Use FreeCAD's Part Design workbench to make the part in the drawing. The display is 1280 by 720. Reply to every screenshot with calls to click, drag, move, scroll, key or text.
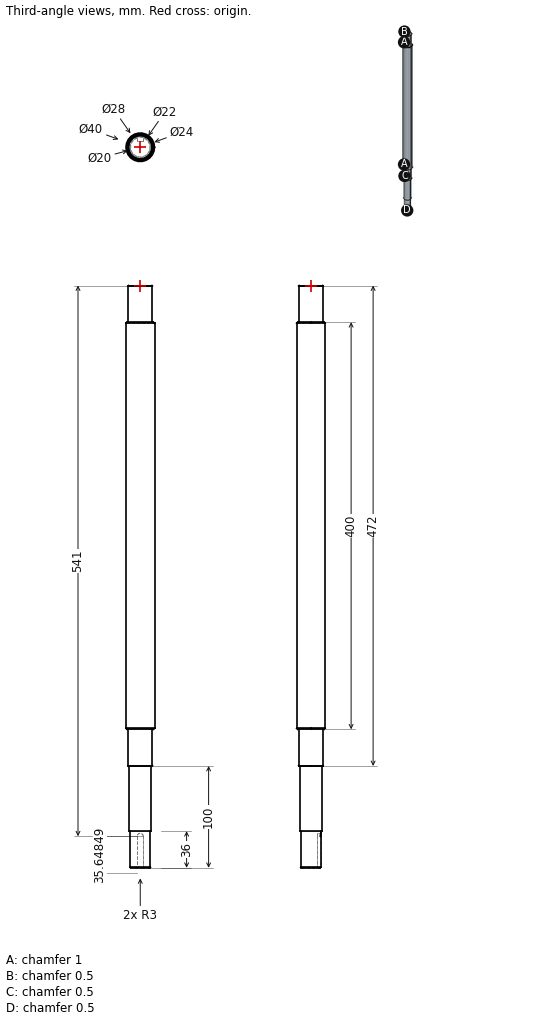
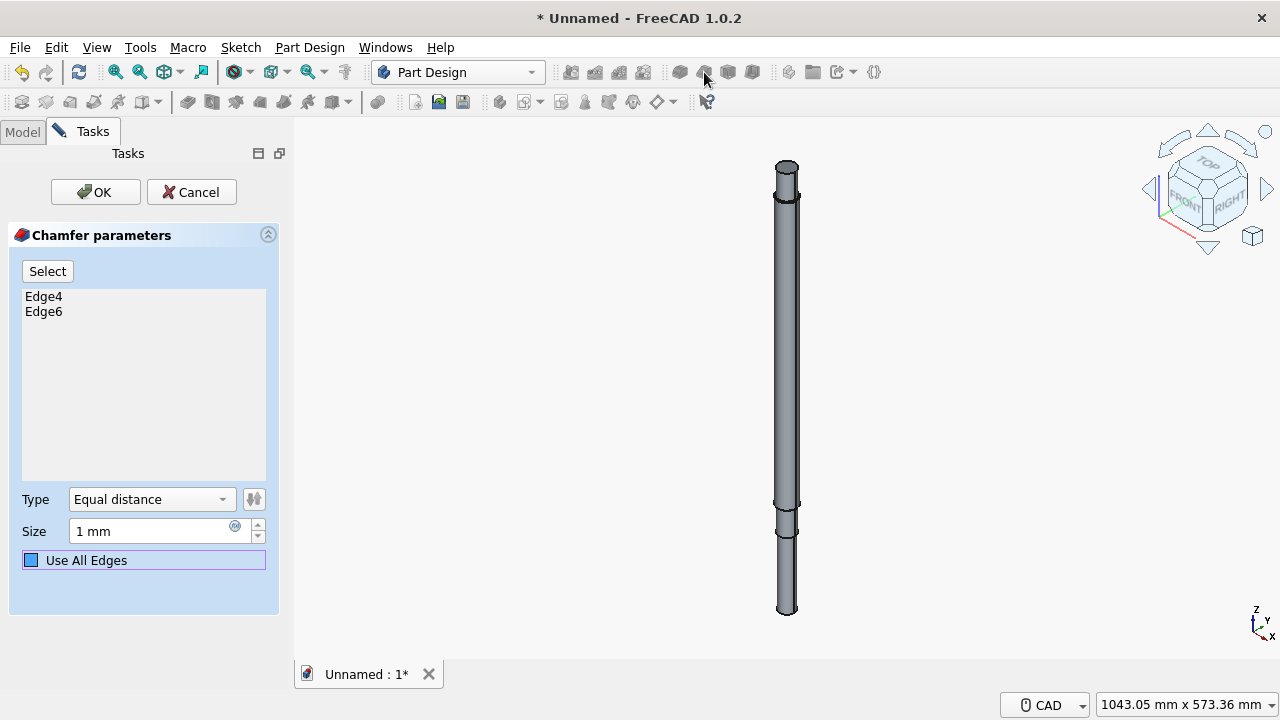
click(96, 192)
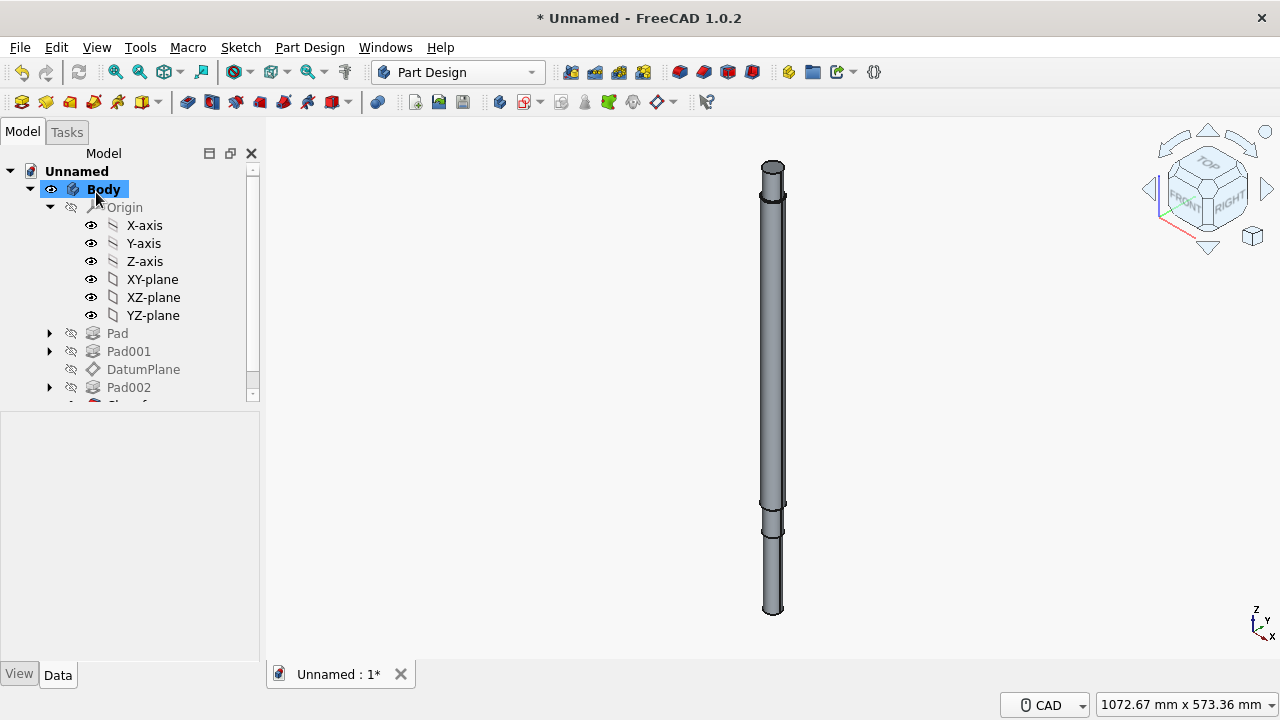
click(762, 165)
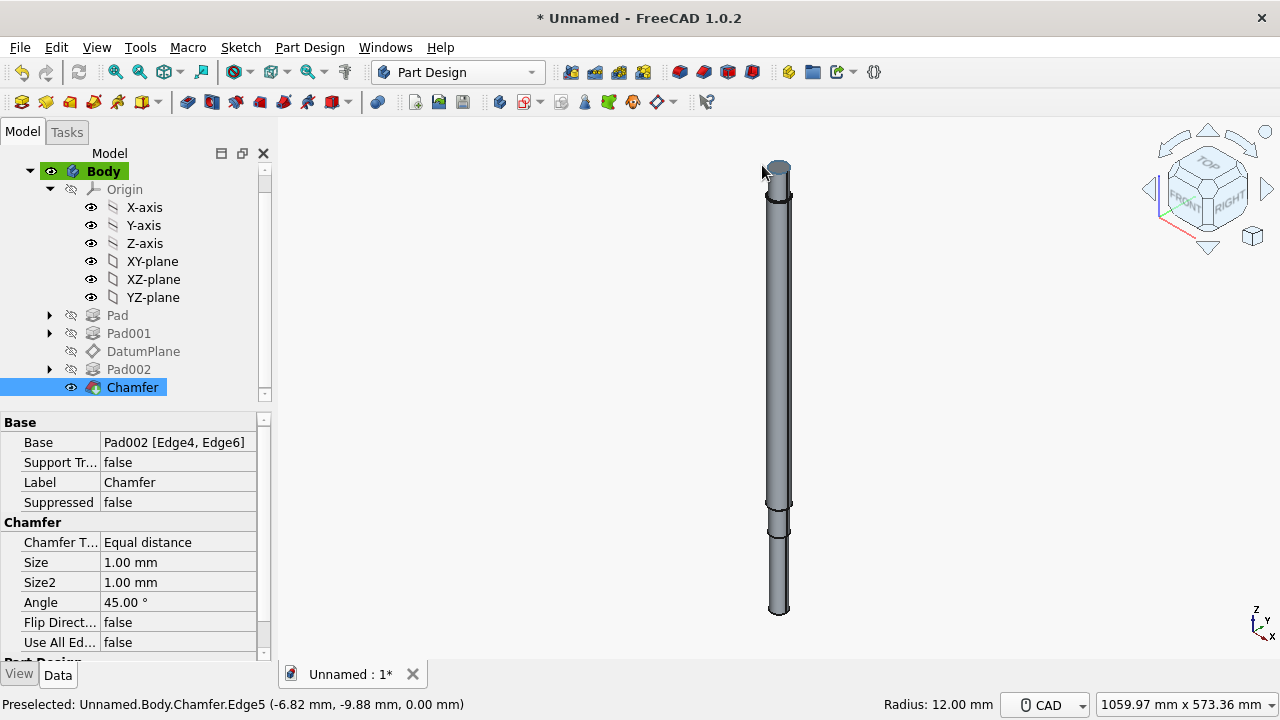
click(704, 72)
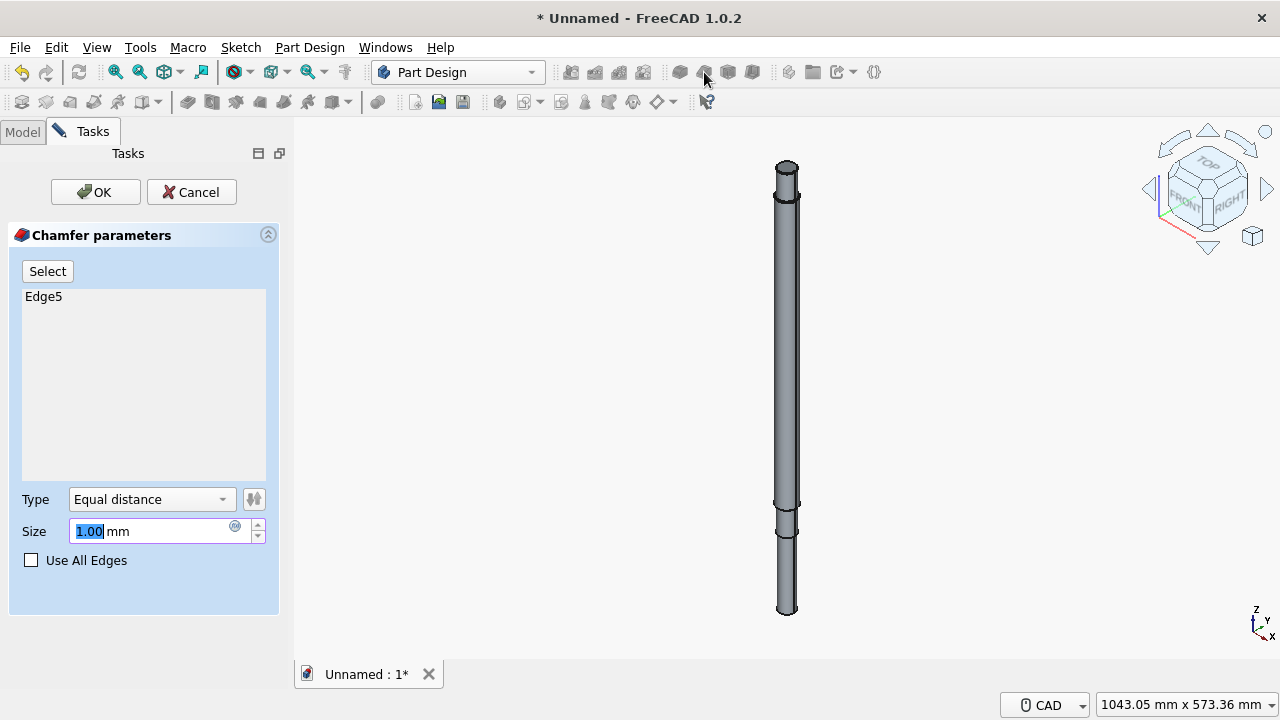
text(0.5)
key(Tab)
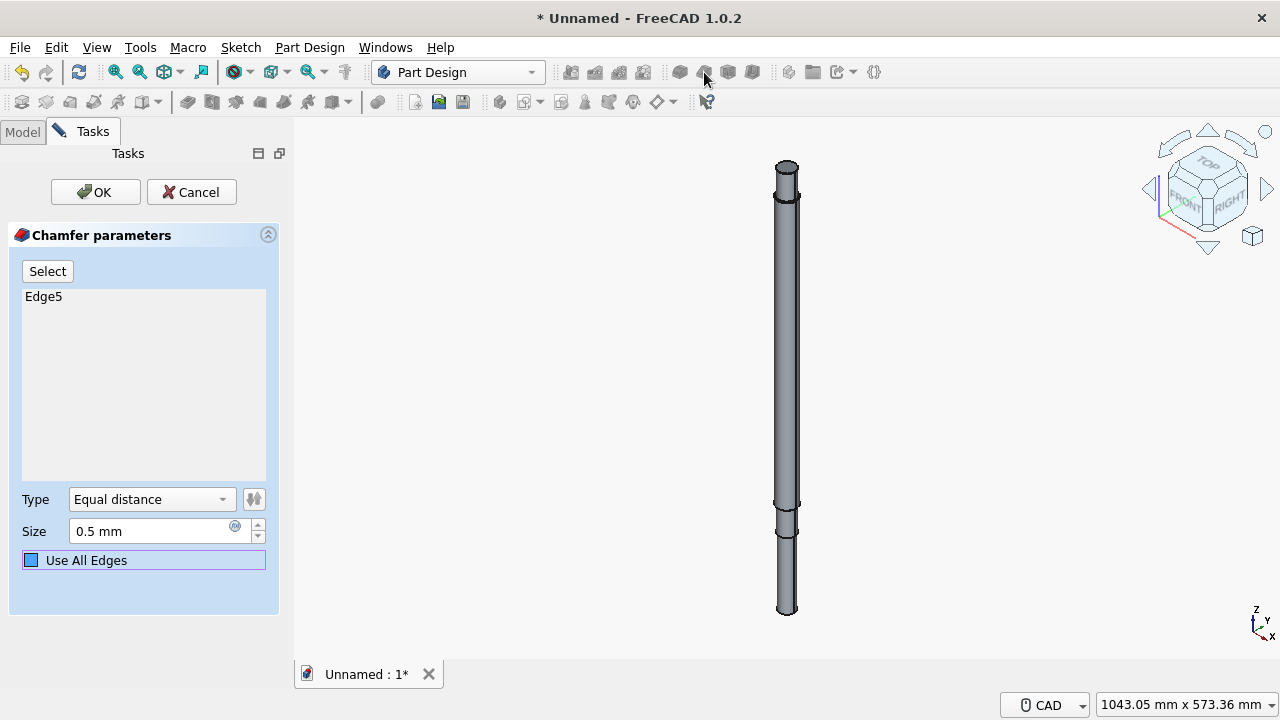
click(96, 192)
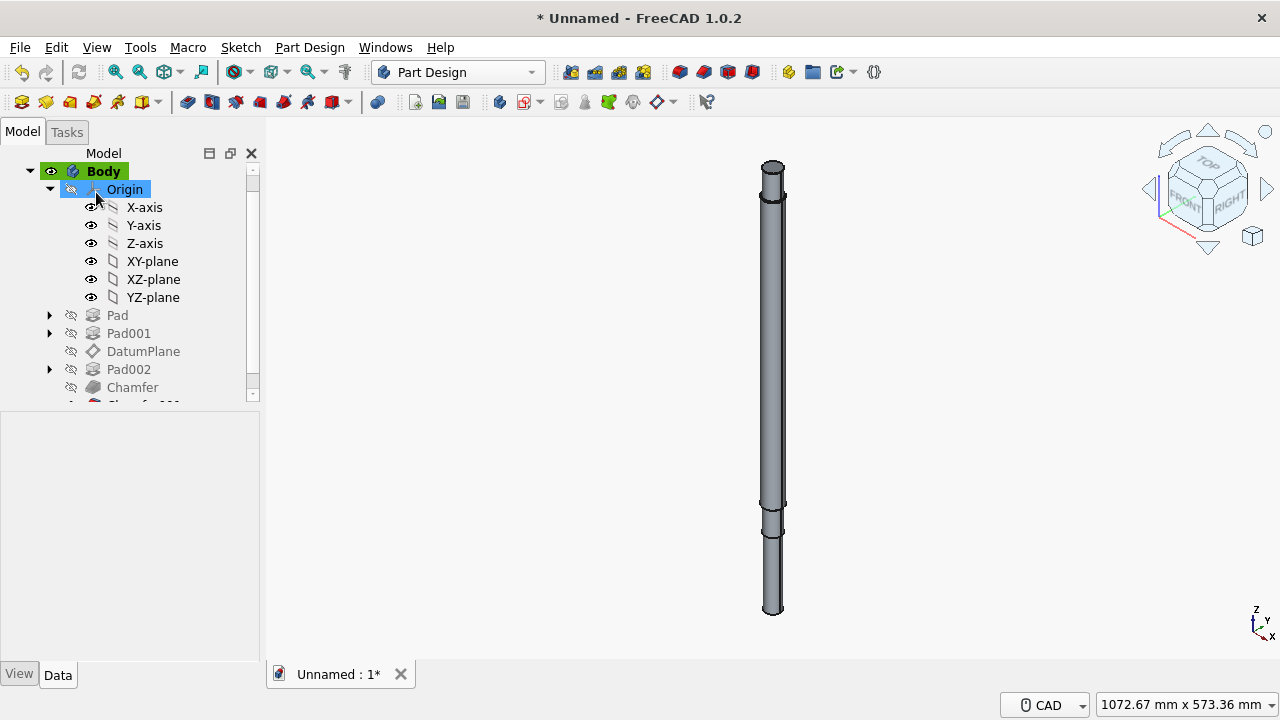
click(763, 534)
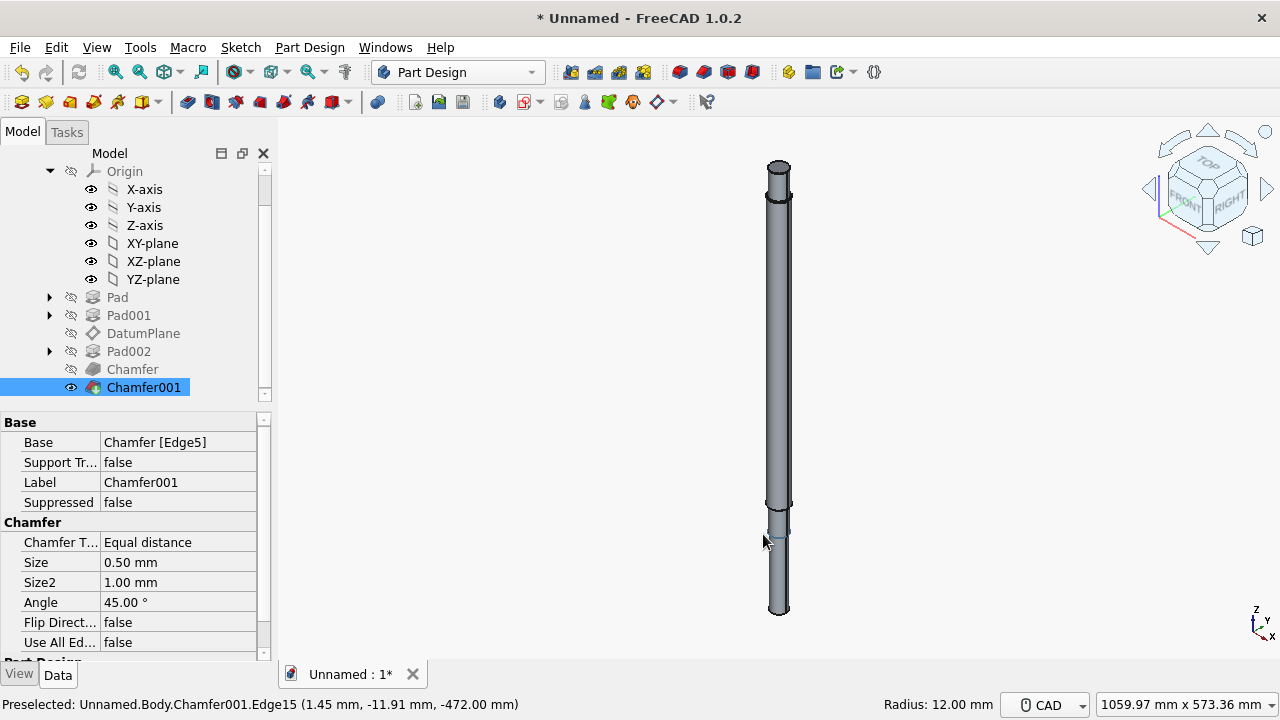
click(704, 72)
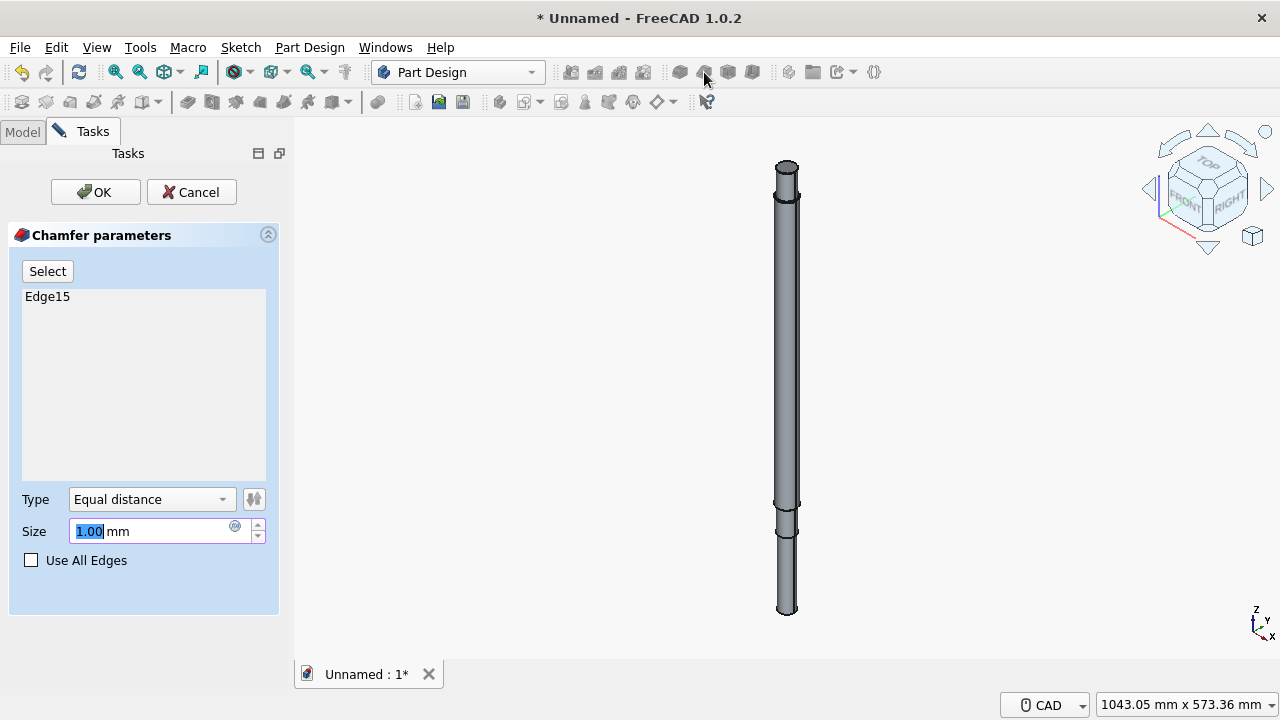
text(0.5)
key(Tab)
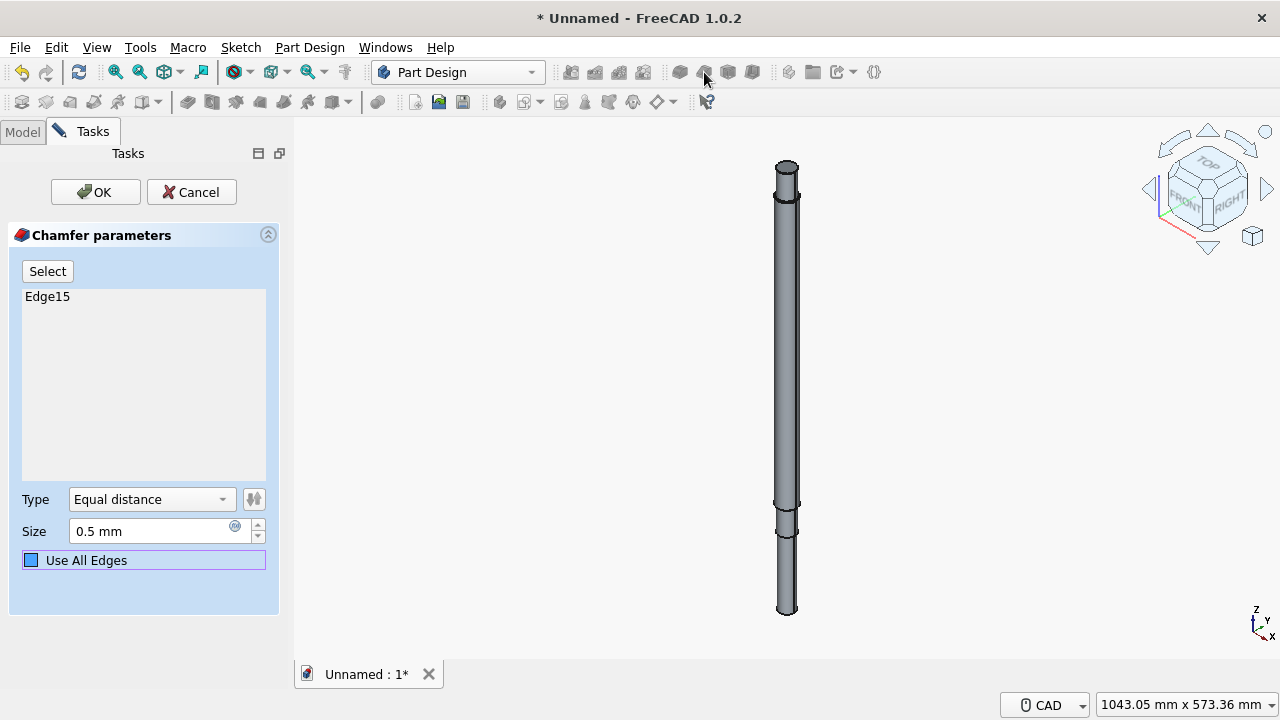
click(96, 192)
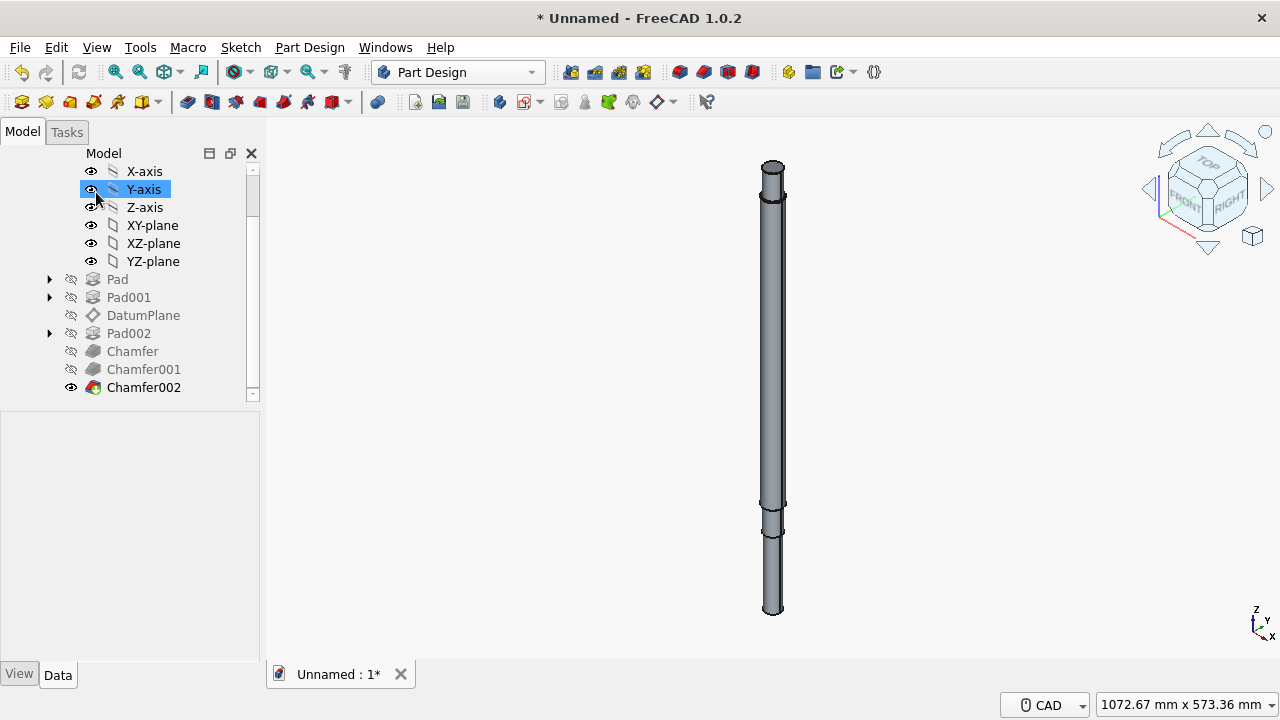
key(5)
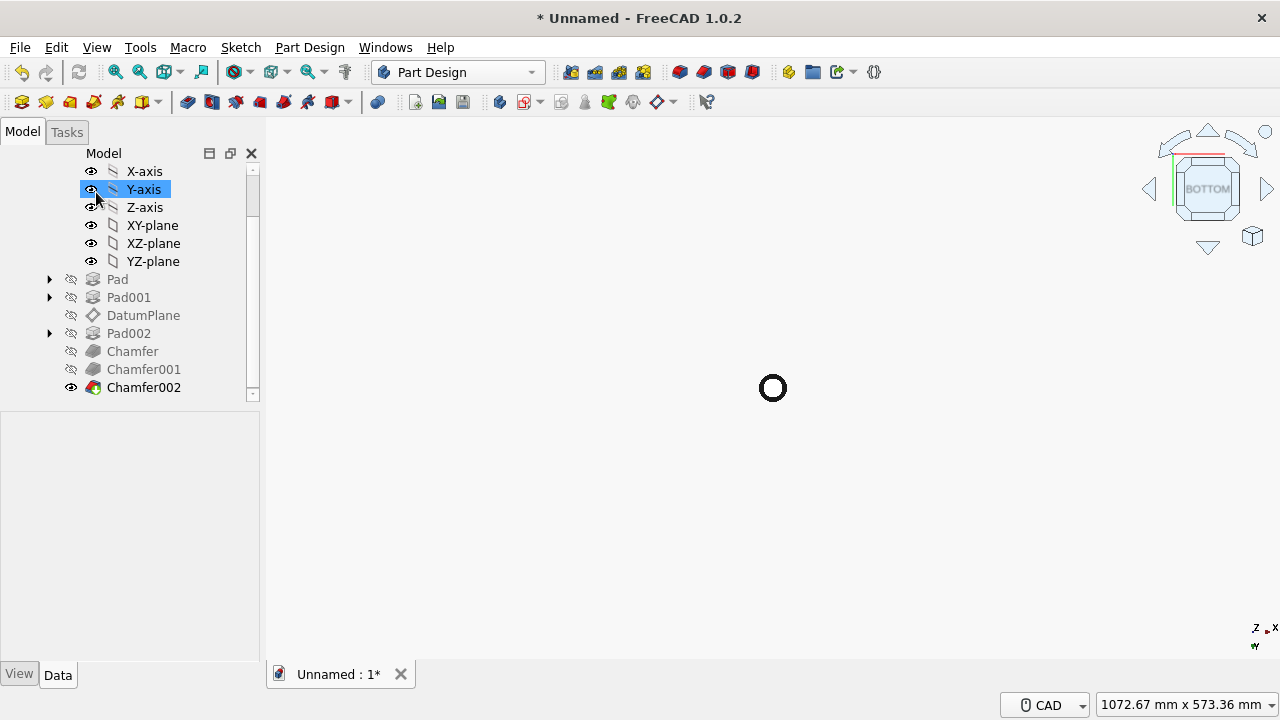
click(116, 72)